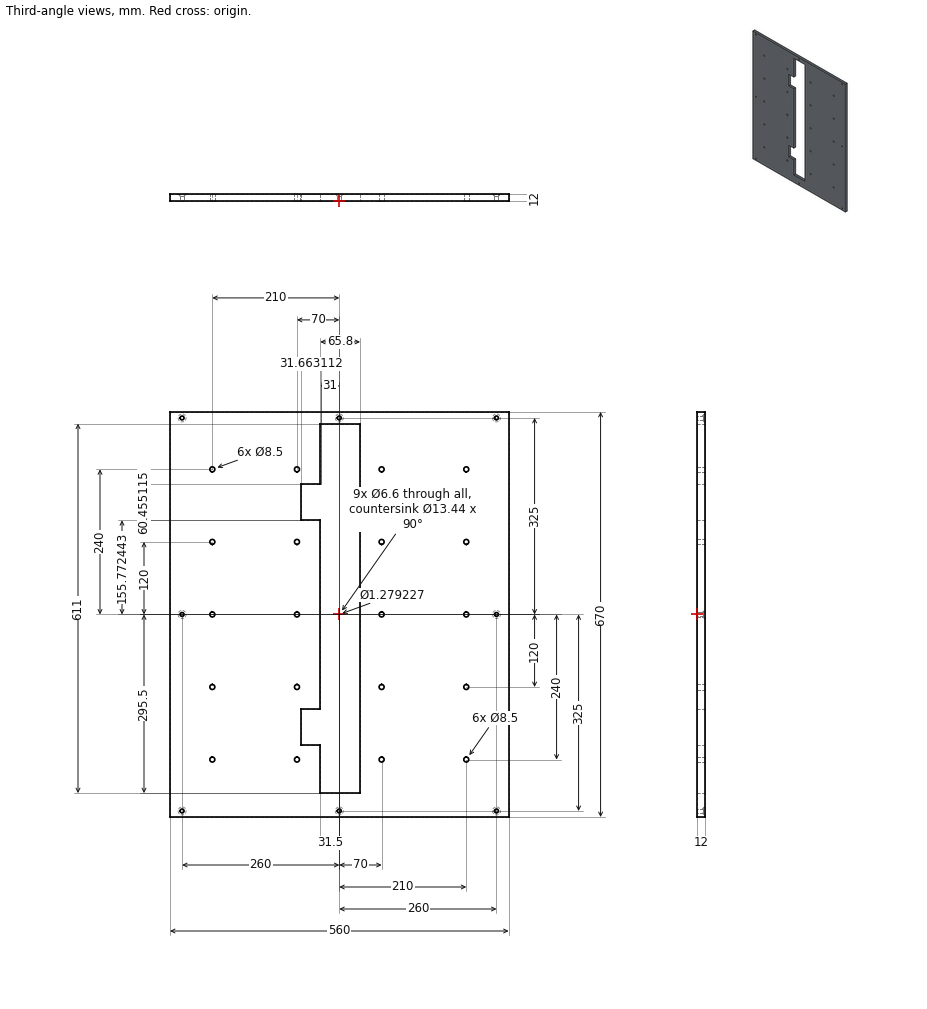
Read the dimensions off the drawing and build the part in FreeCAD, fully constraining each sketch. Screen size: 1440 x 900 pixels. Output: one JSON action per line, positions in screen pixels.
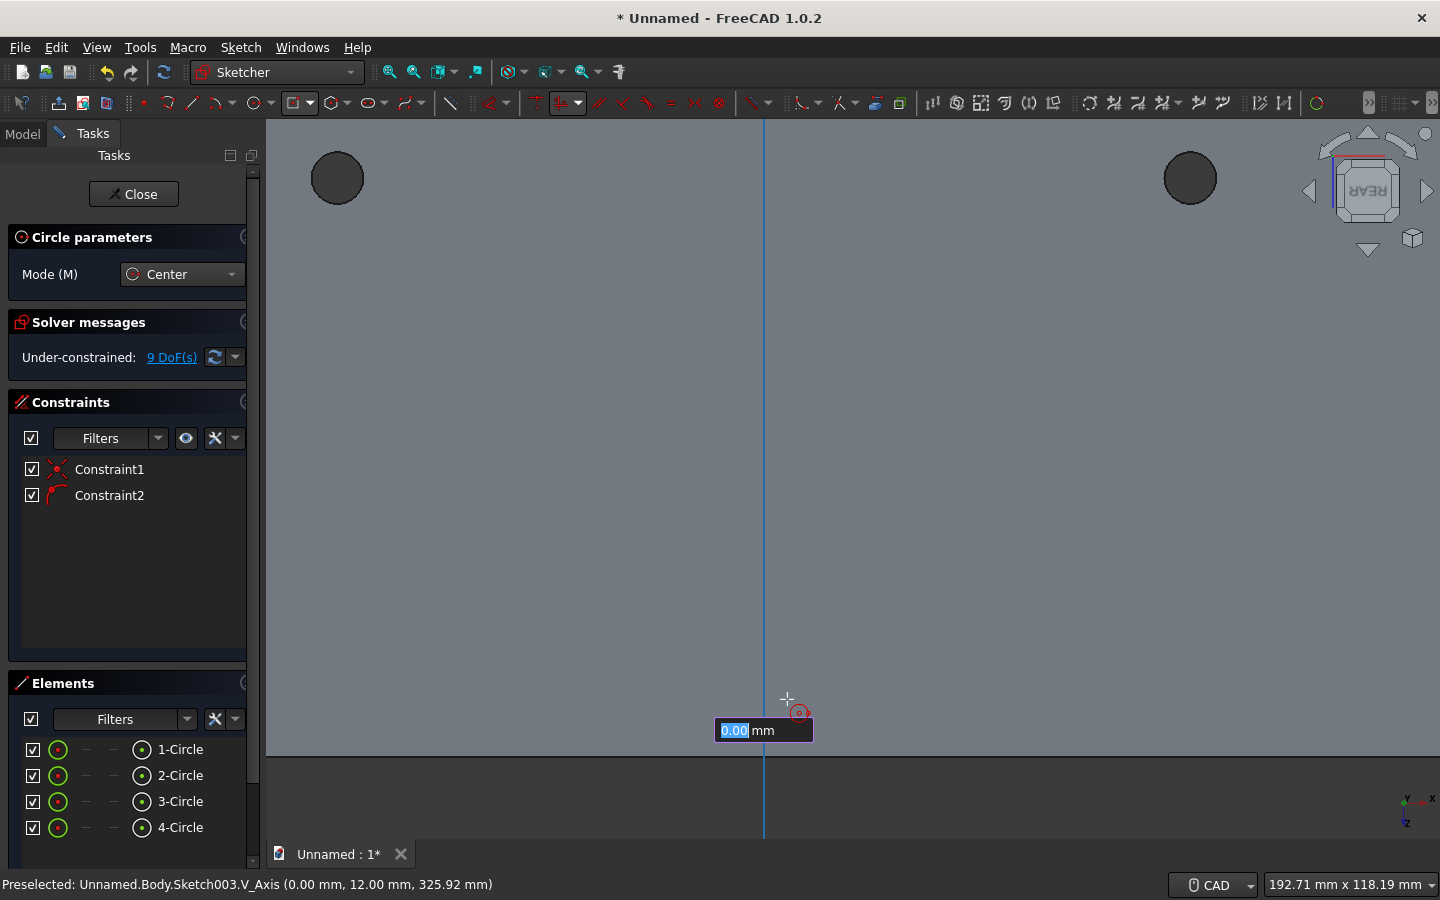
{"action": "left_click", "coordinate": [783, 689]}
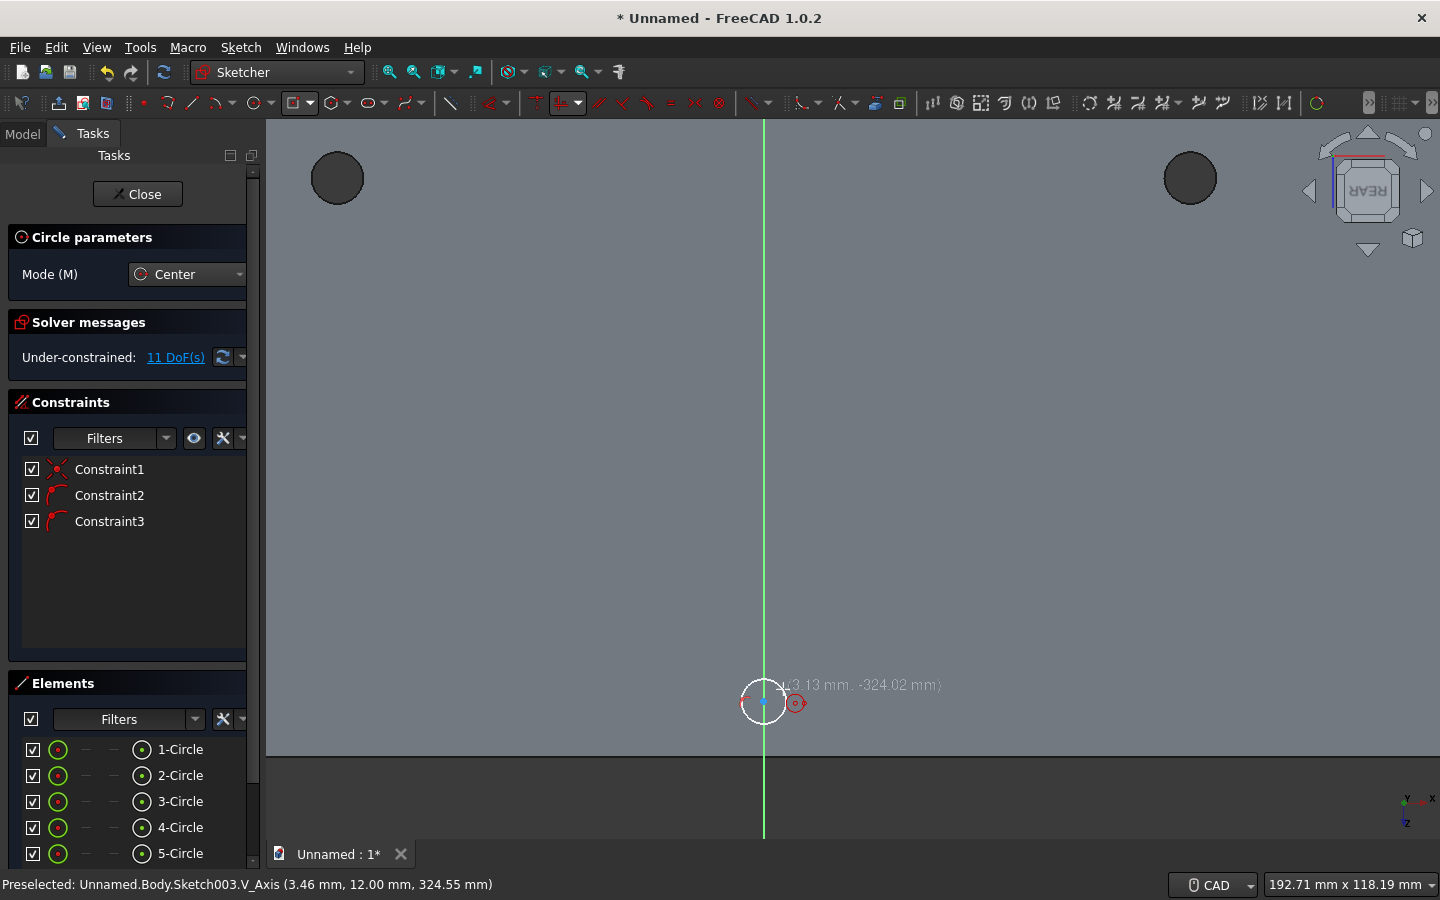
{"action": "scroll", "coordinate": [787, 699], "scroll_direction": "down", "scroll_amount": 11}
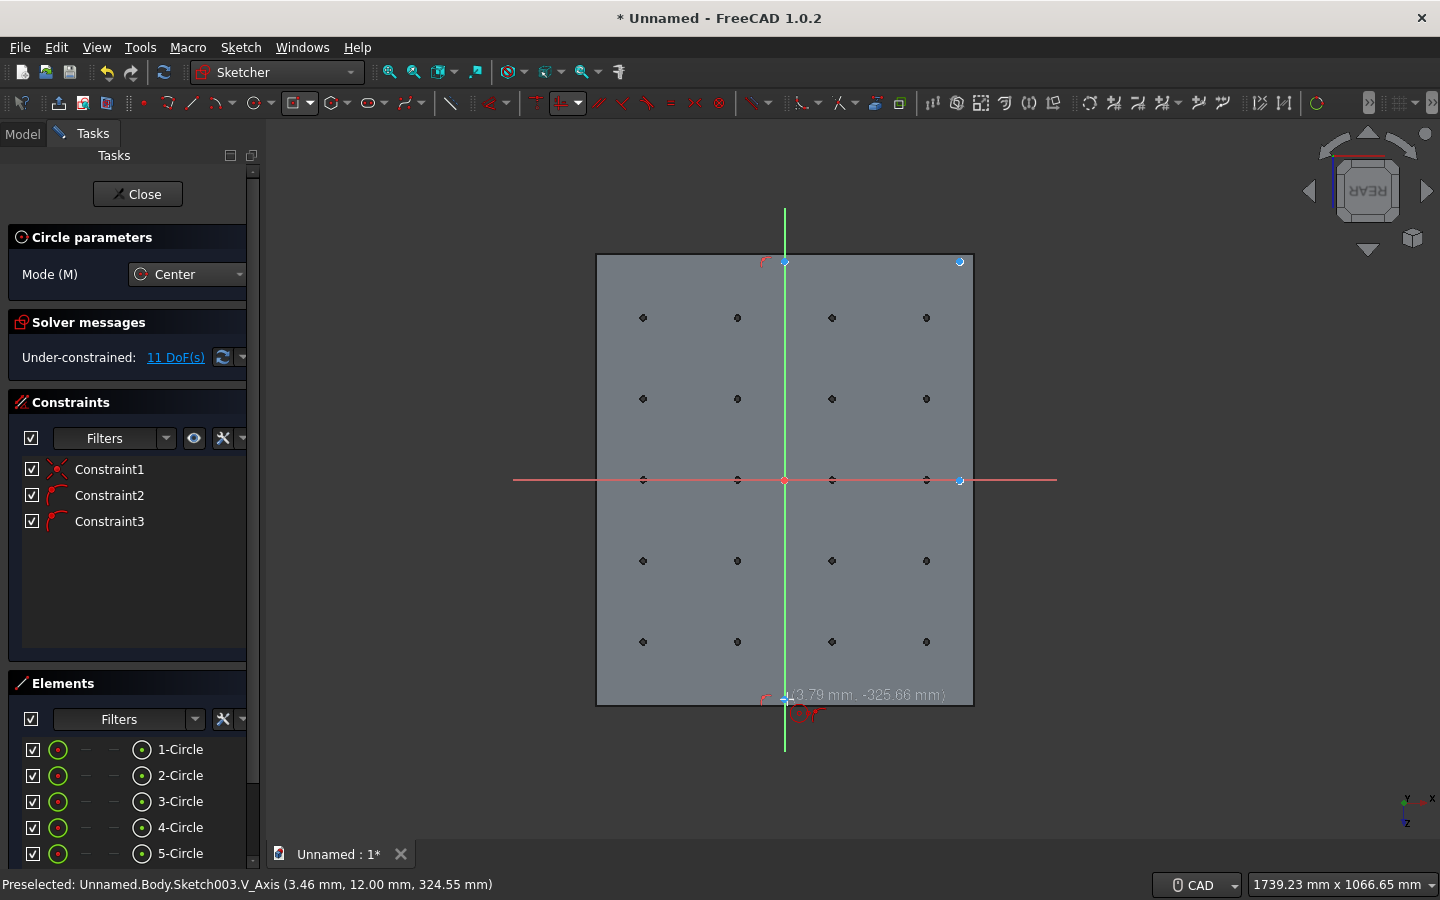
{"action": "scroll", "coordinate": [609, 480], "scroll_direction": "up", "scroll_amount": 12}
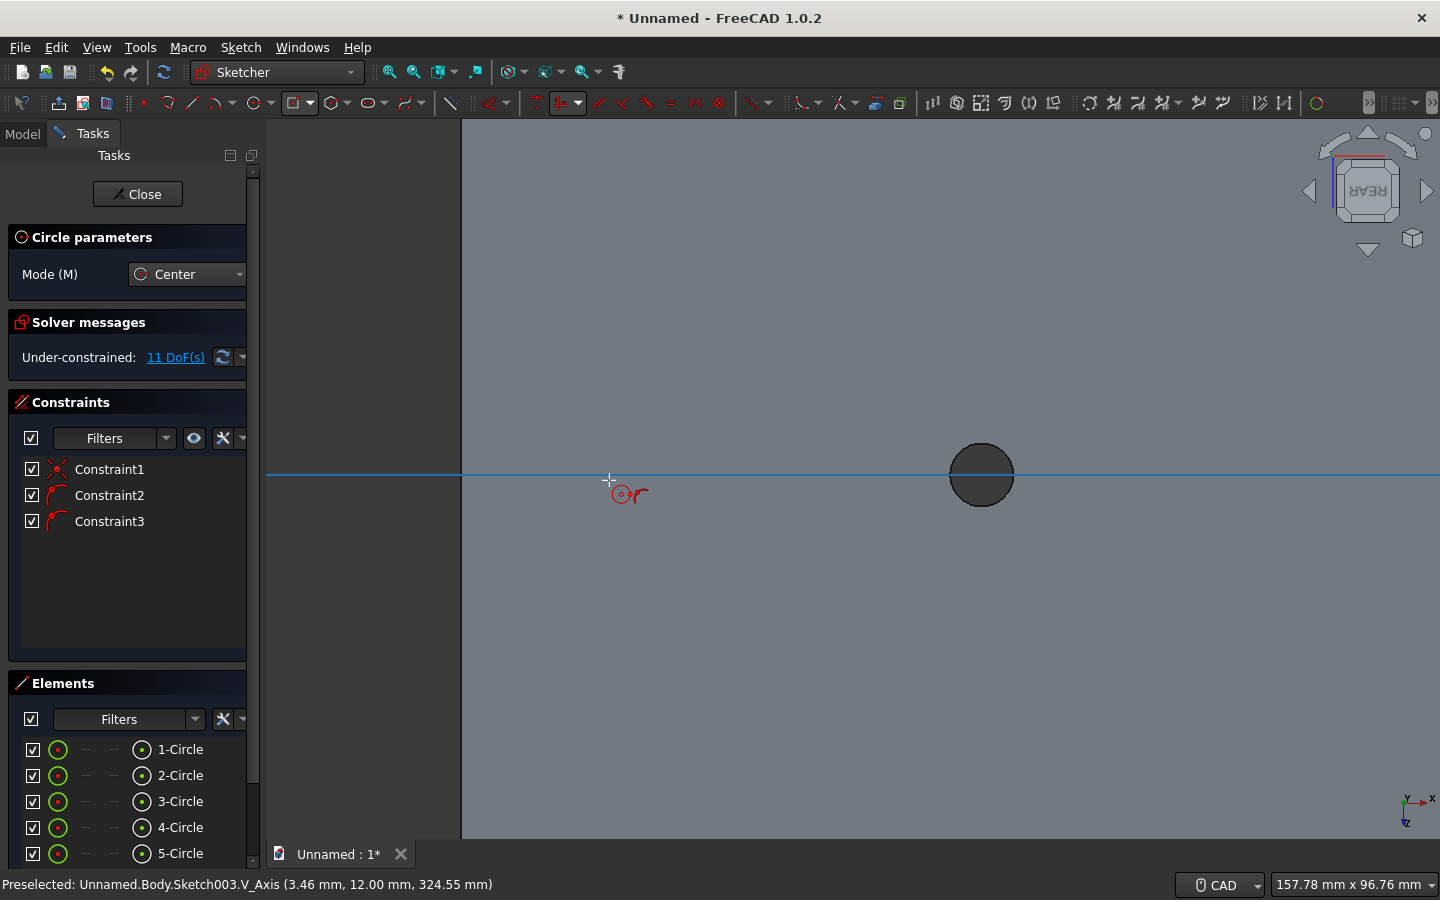
{"action": "scroll", "coordinate": [609, 479], "scroll_direction": "down", "scroll_amount": 12}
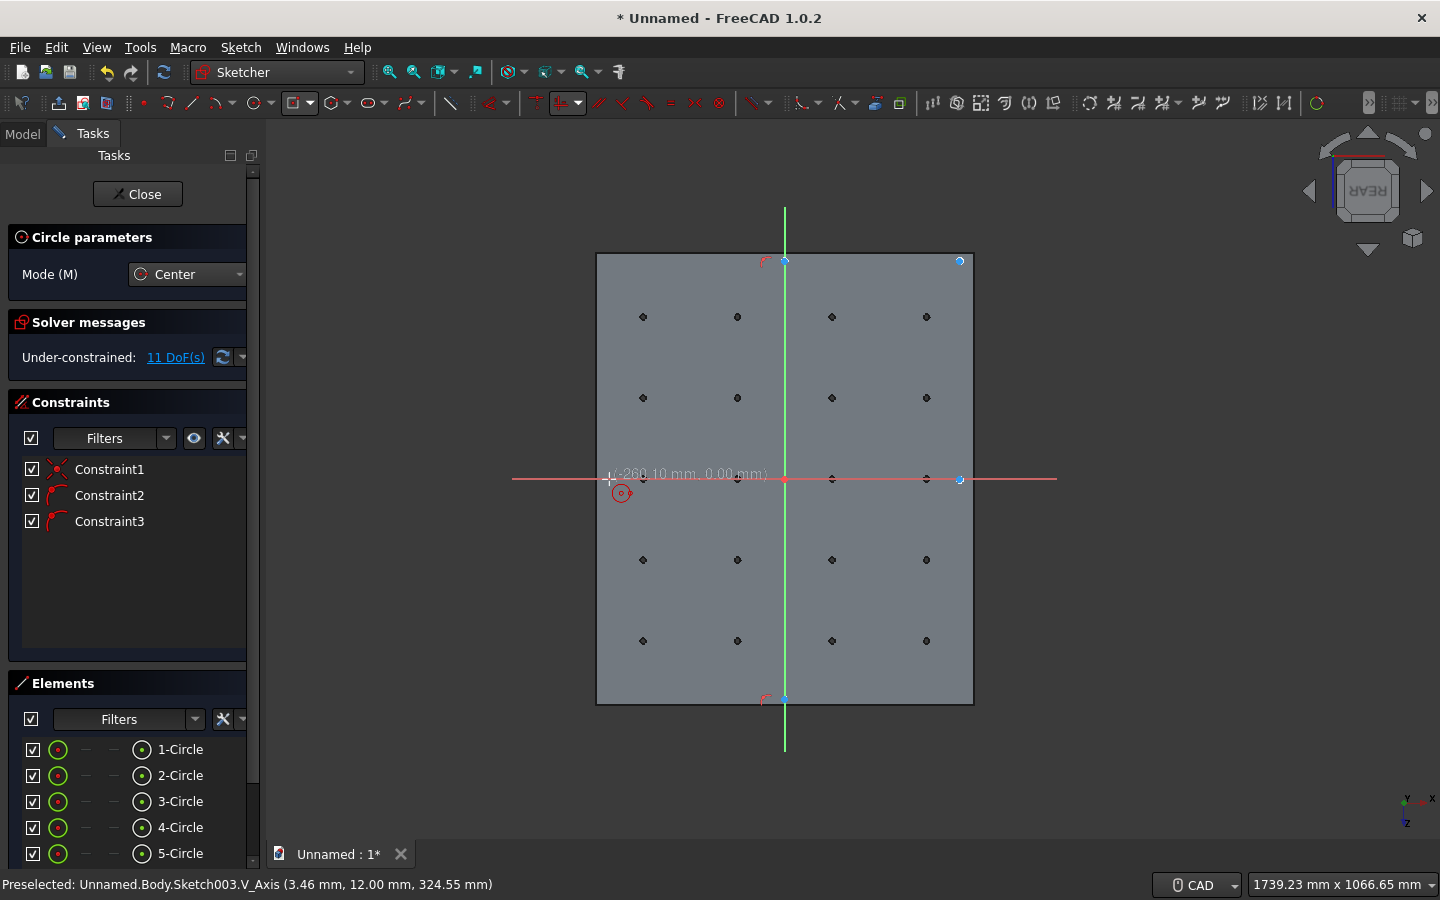
{"action": "left_click", "coordinate": [609, 479]}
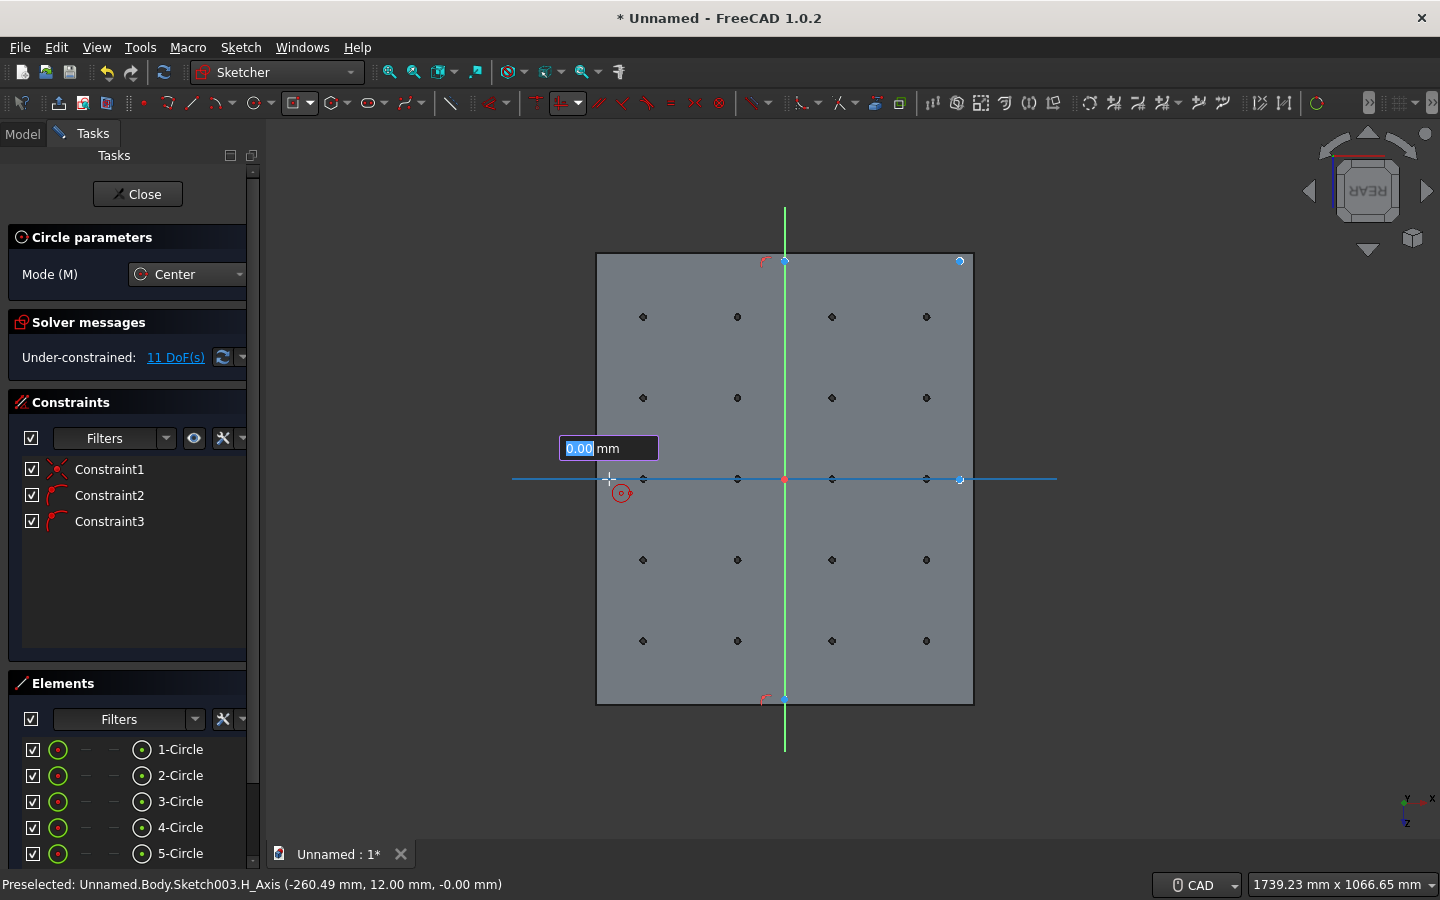
{"action": "scroll", "coordinate": [609, 481], "scroll_direction": "up", "scroll_amount": 11}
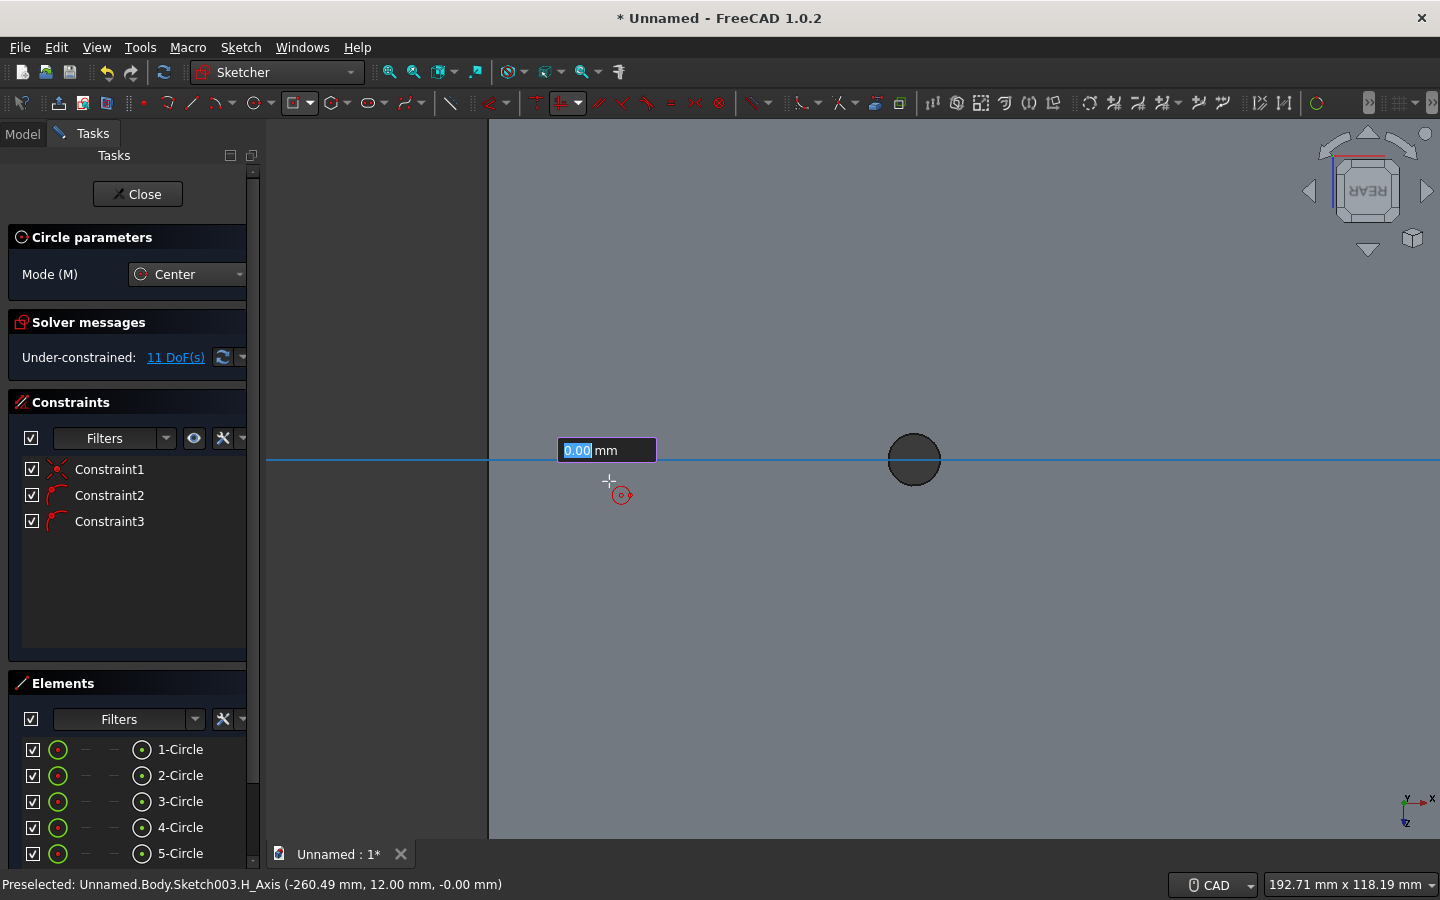
{"action": "left_click", "coordinate": [603, 479]}